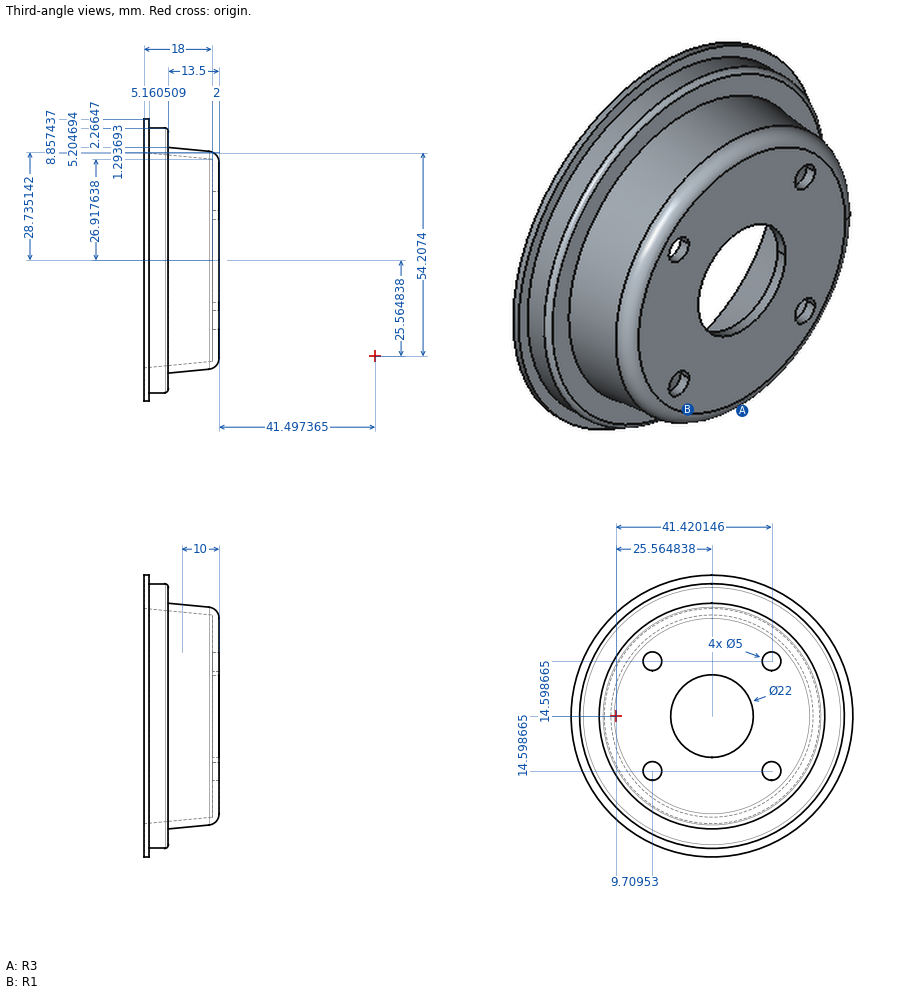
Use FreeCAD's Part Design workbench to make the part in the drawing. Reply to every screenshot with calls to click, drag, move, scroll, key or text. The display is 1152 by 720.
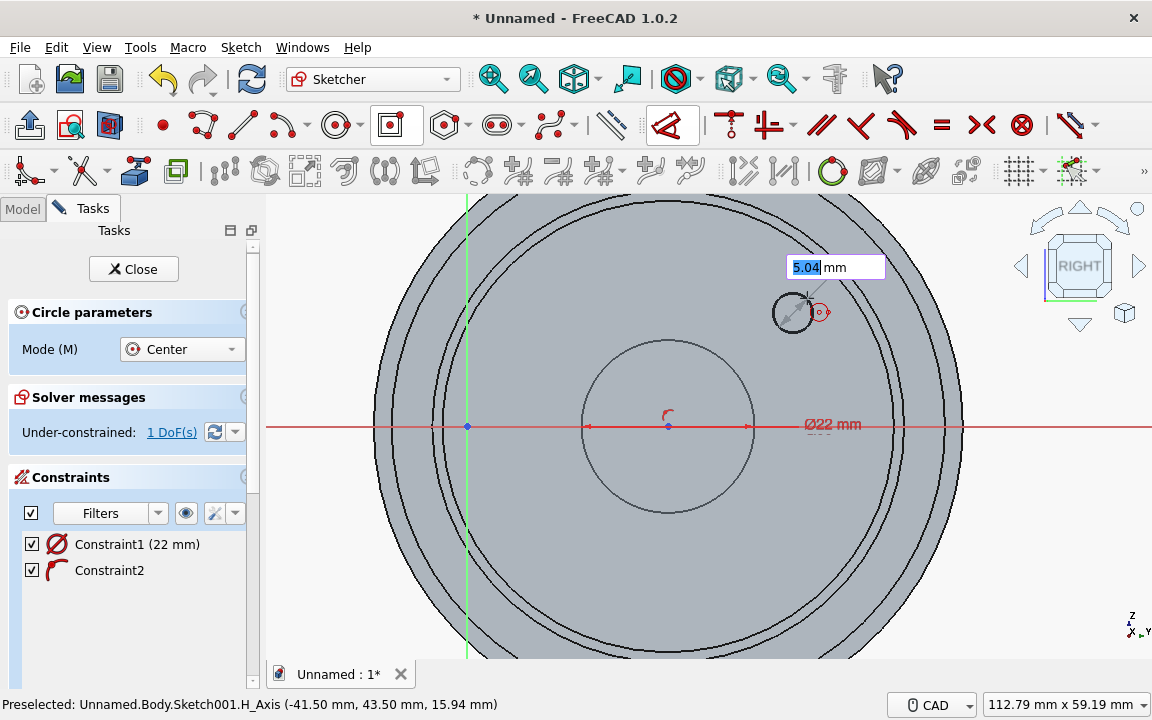
text(5)
key(Return)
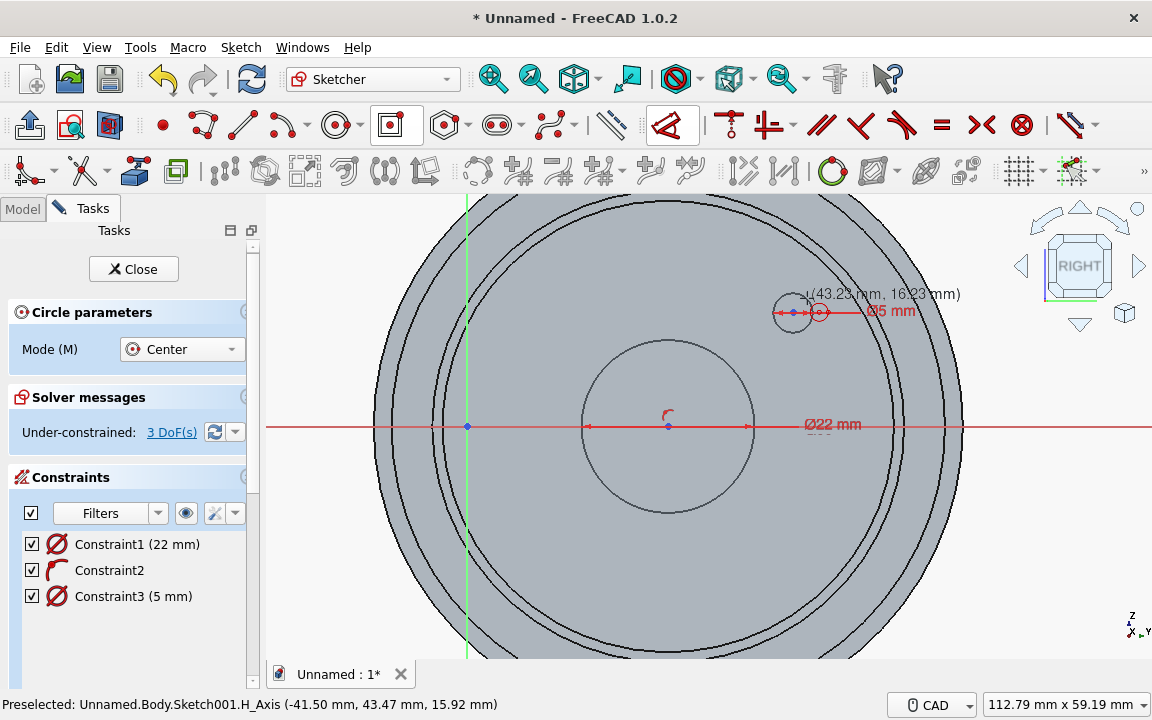
click(793, 541)
move(807, 527)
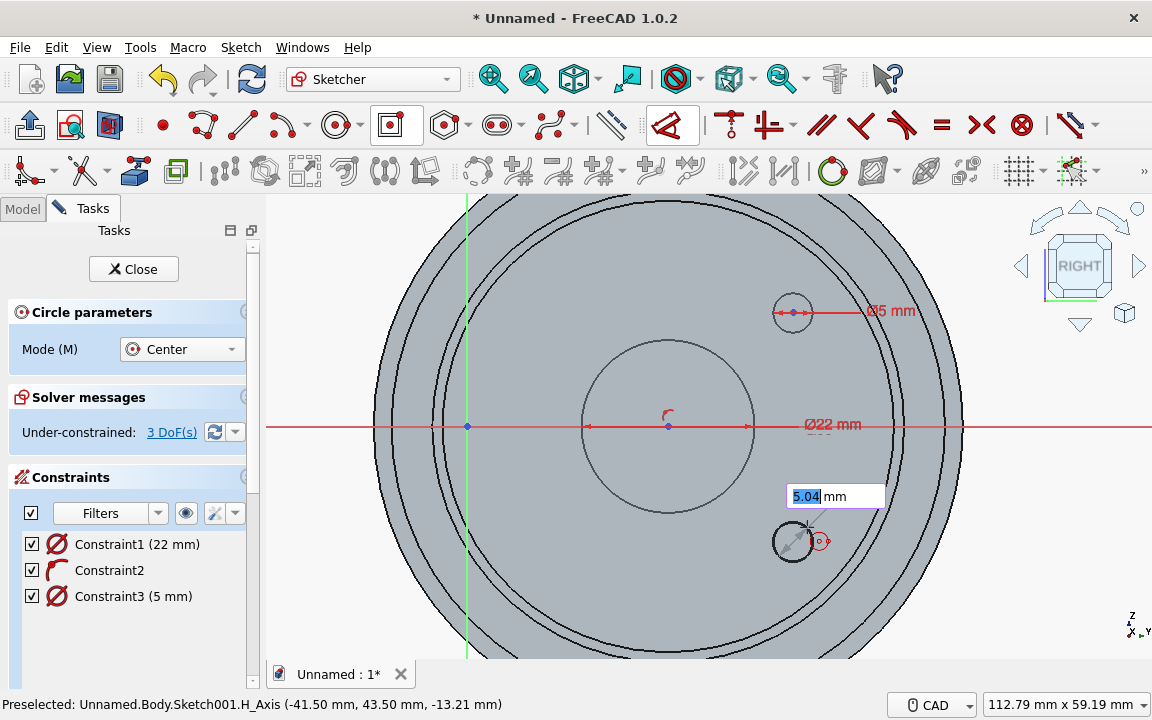
text(5)
key(Return)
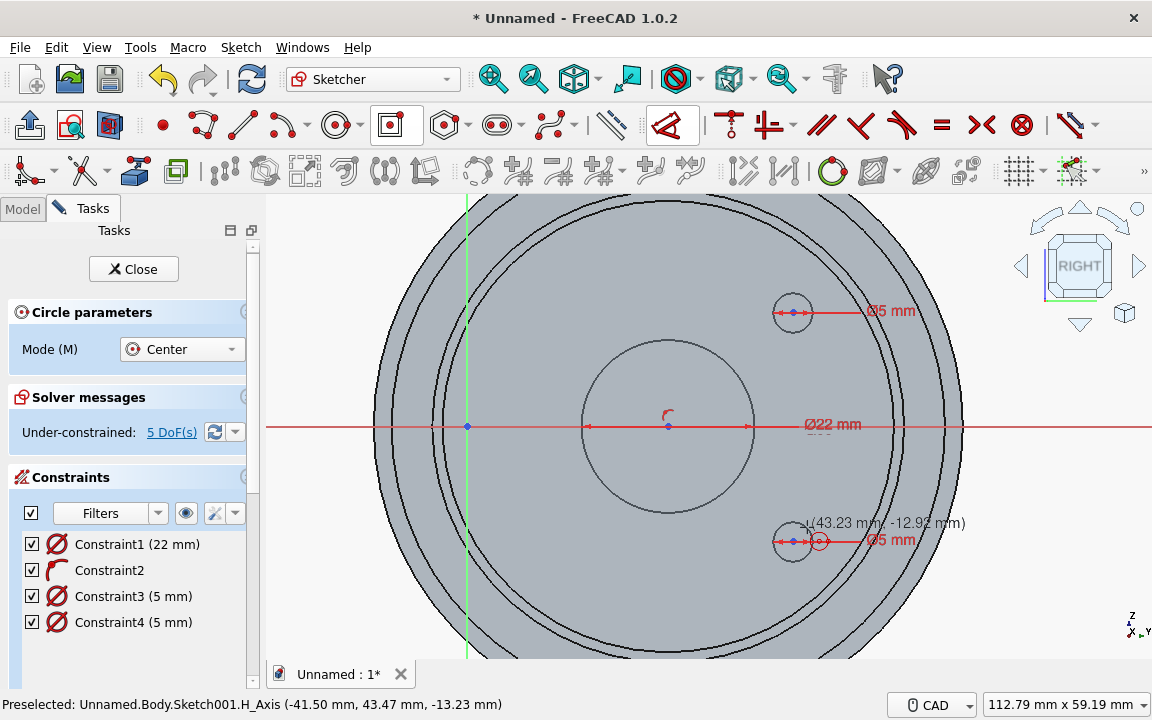
click(544, 541)
move(558, 527)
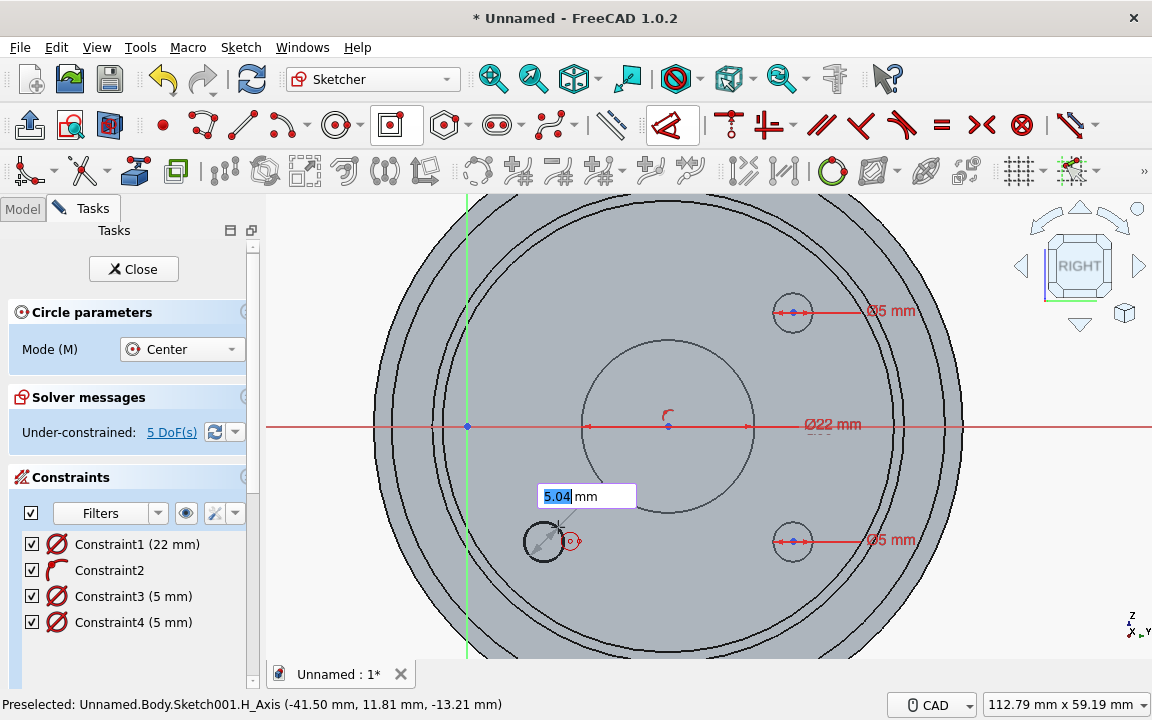
text(5)
key(Return)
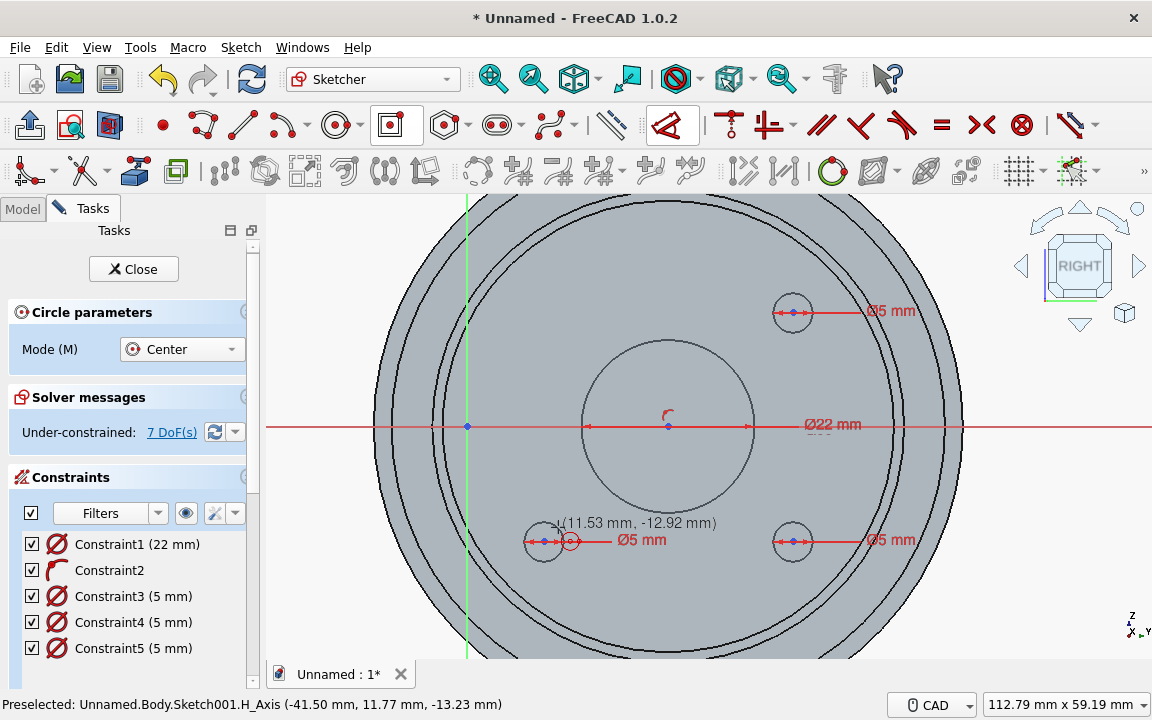
click(544, 312)
move(558, 298)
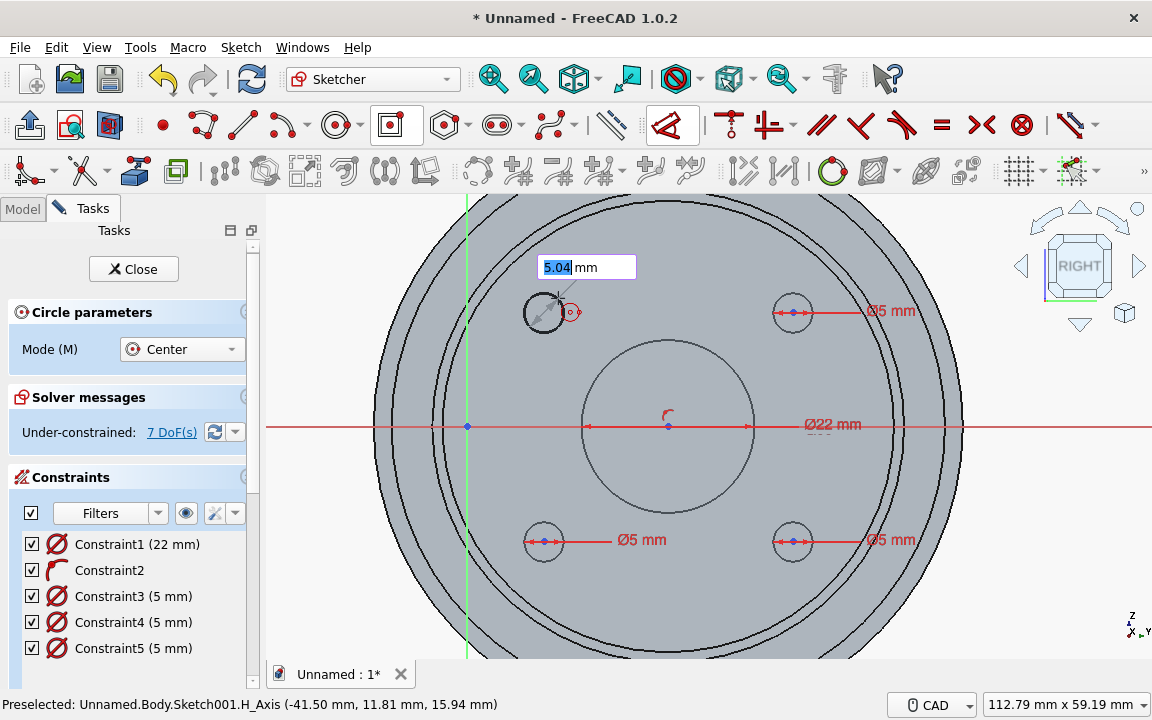
text(5)
key(Return)
key(Escape)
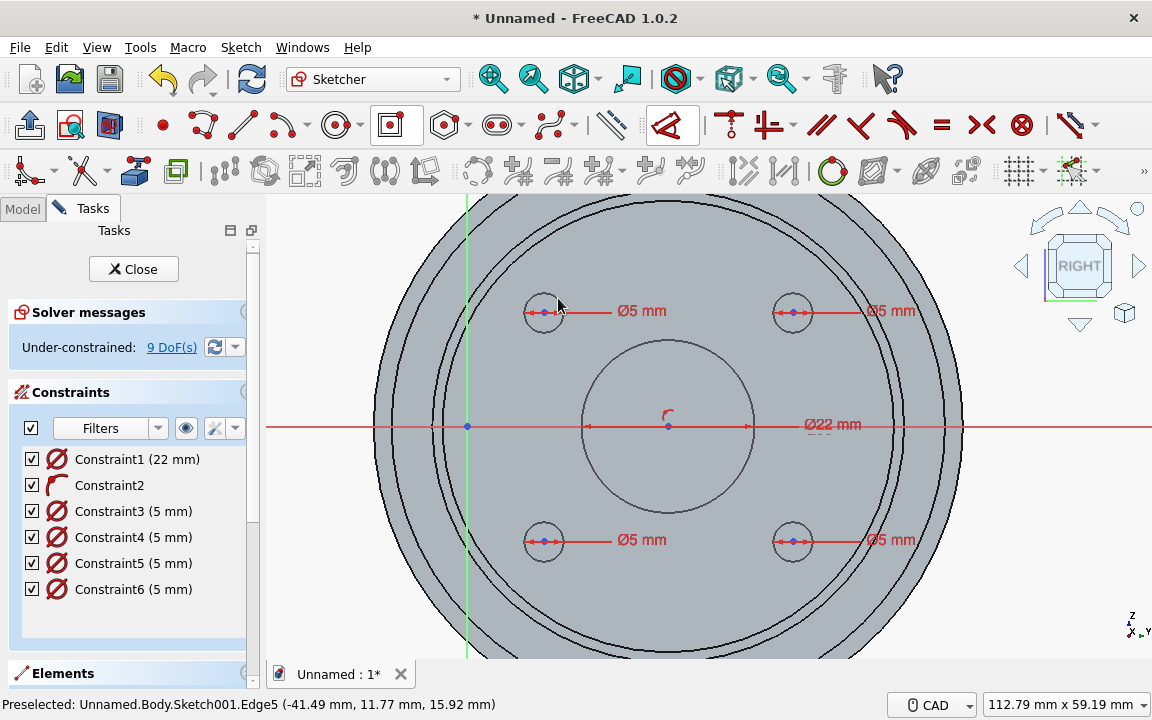
click(544, 542)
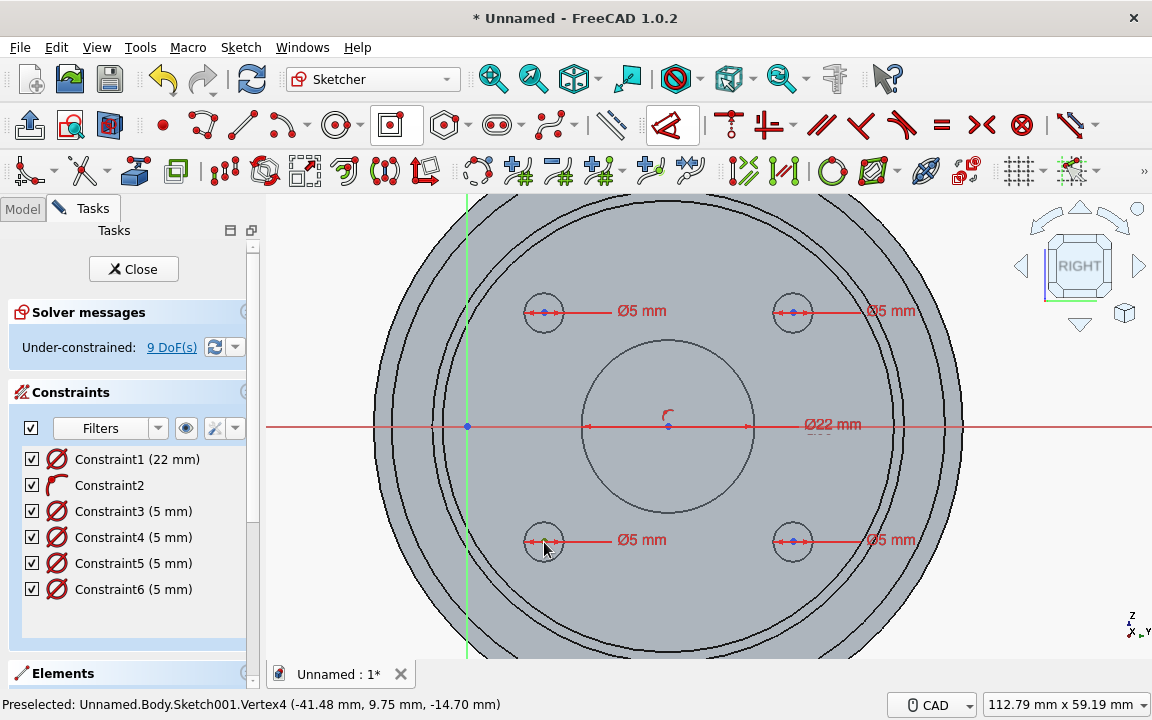
key(l)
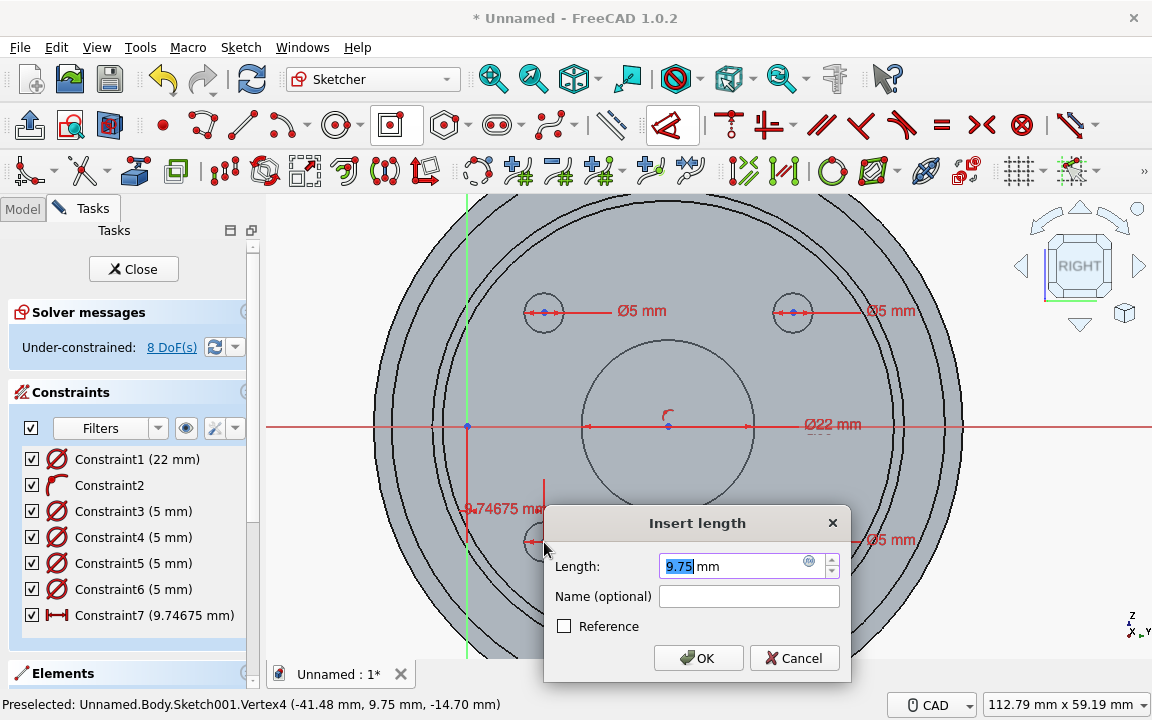
text(9.70953)
key(Return)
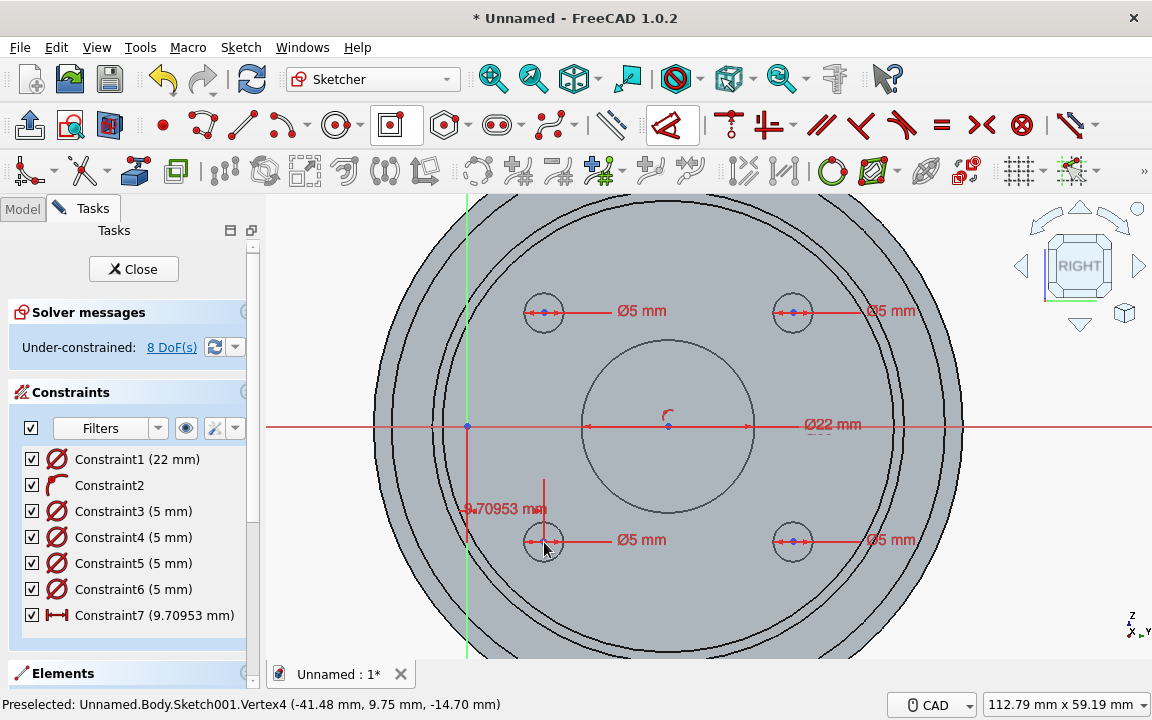
click(544, 313)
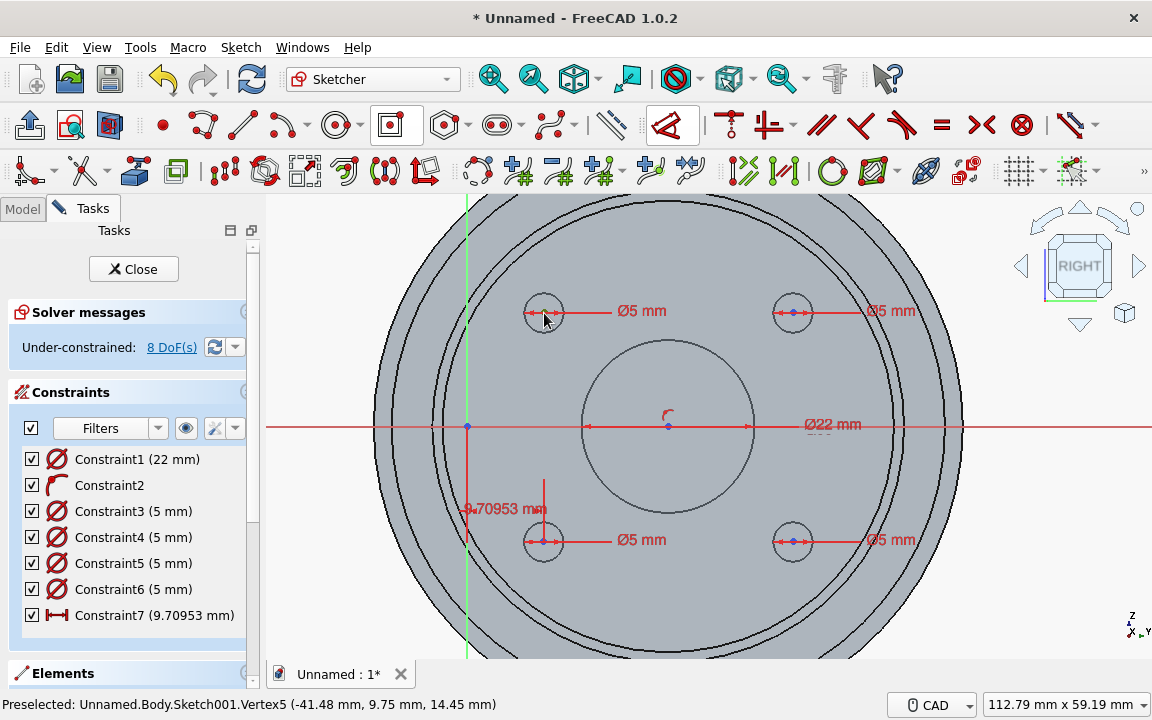
key(l)